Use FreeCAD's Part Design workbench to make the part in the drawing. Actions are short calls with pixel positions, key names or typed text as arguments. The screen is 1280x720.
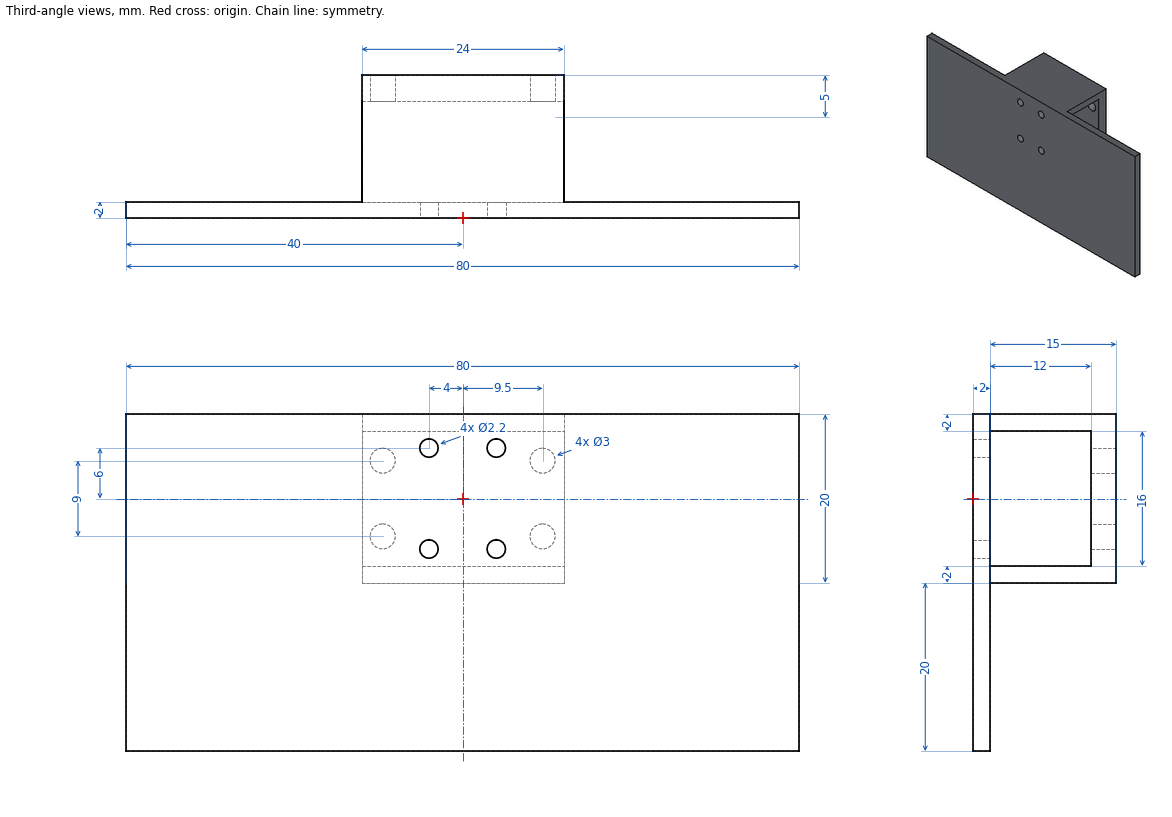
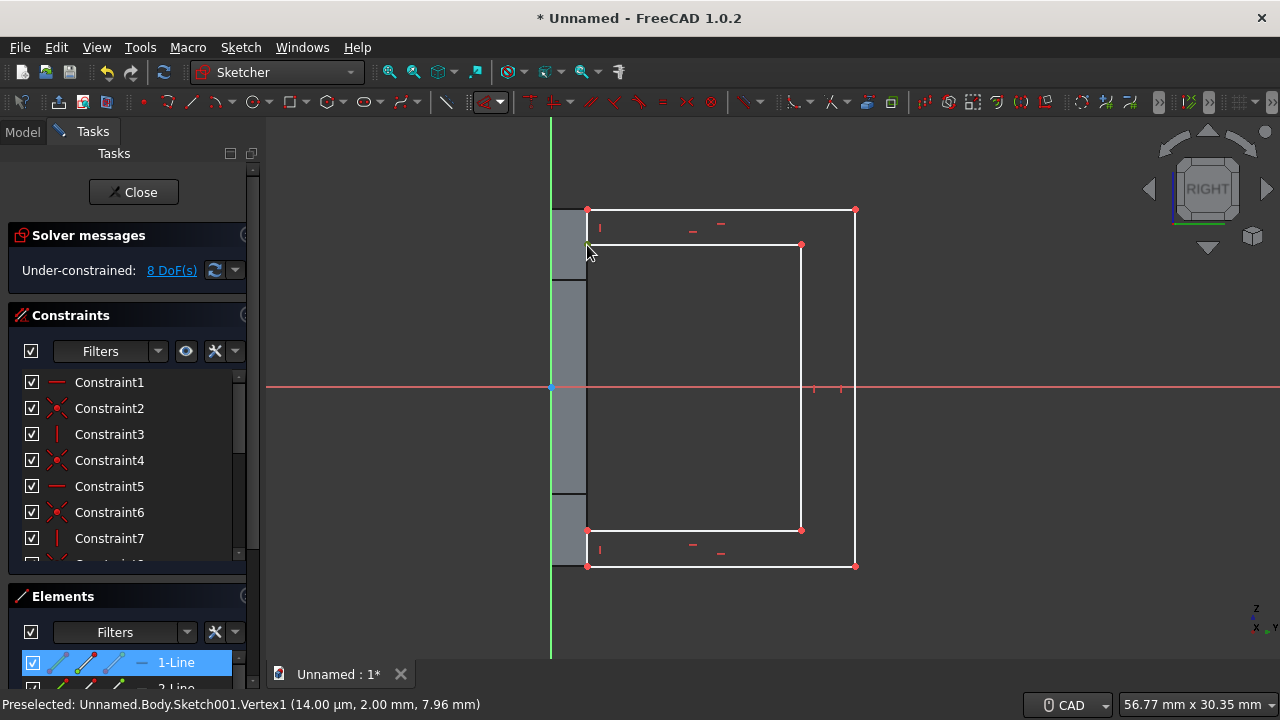
click(587, 531)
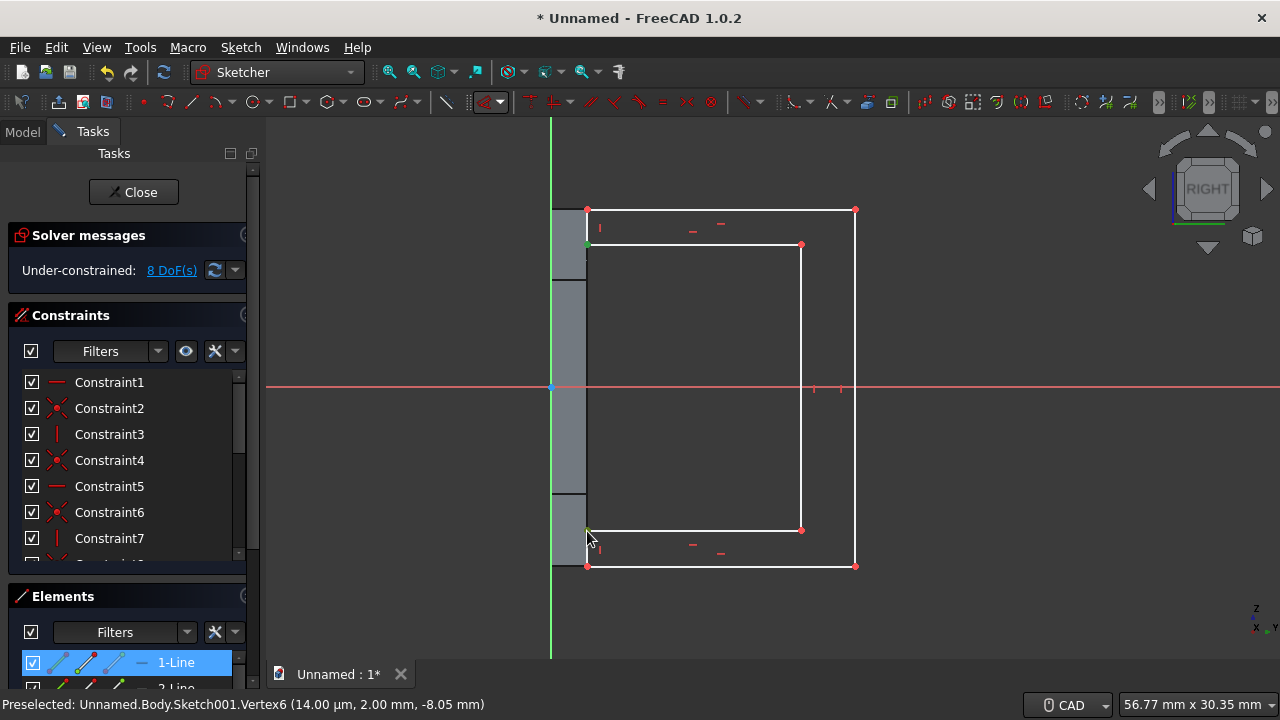
click(353, 387)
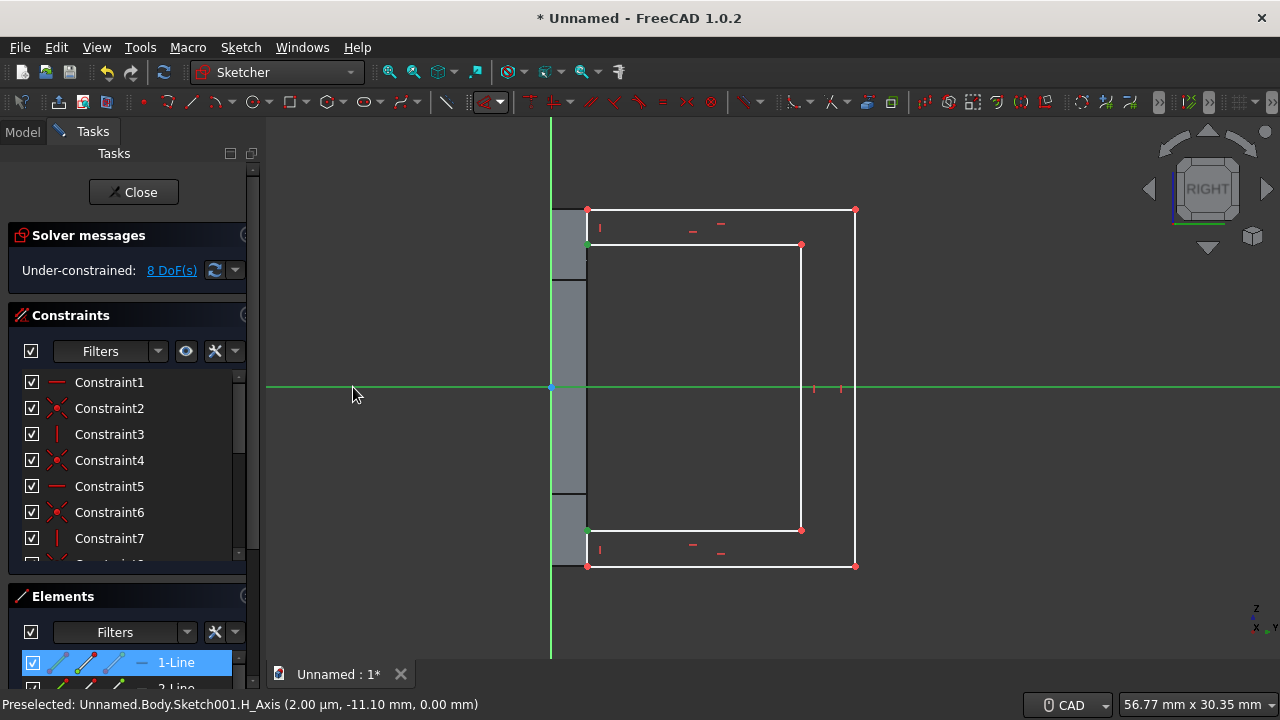
click(688, 102)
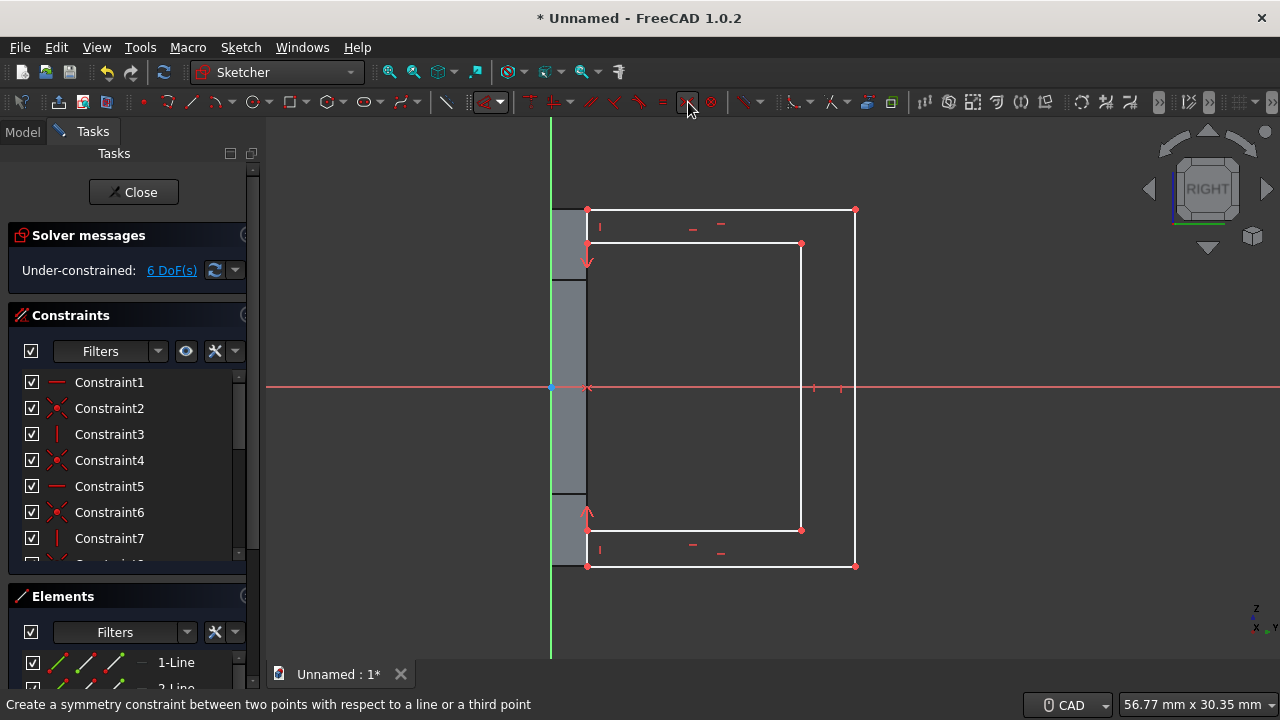
scroll(587, 542, up, 2)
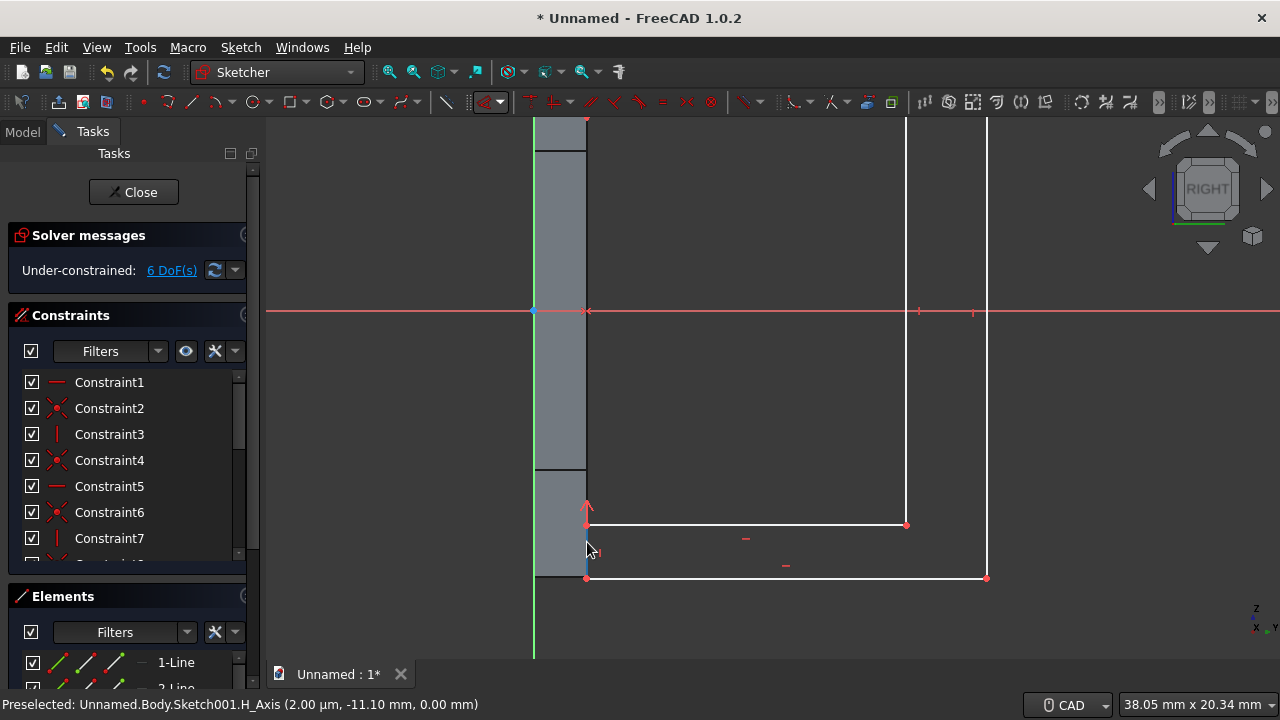
click(587, 541)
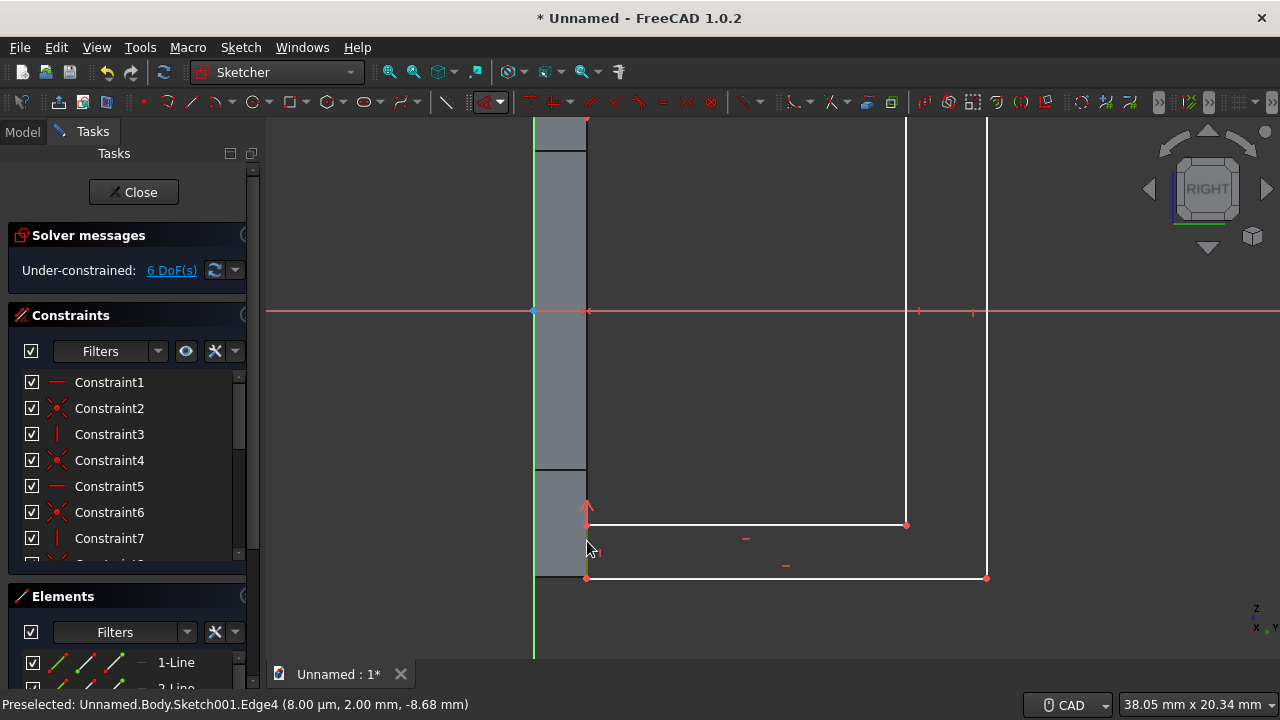
click(502, 102)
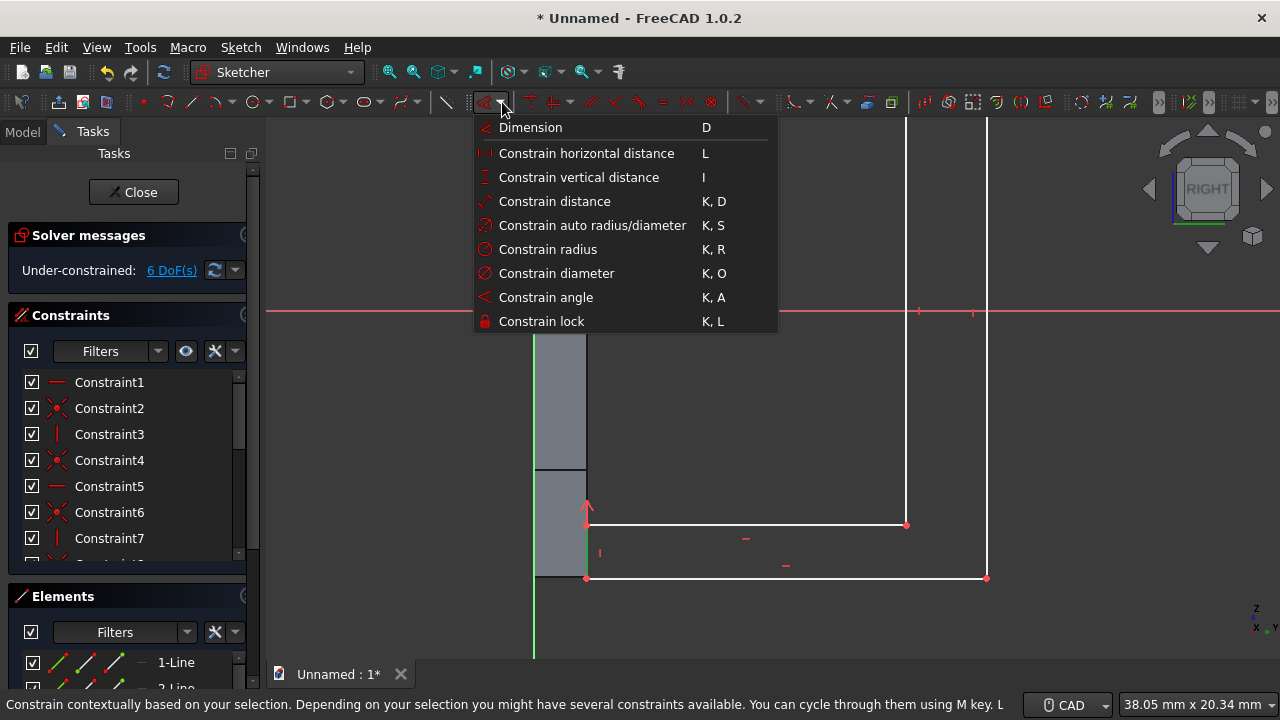
click(626, 177)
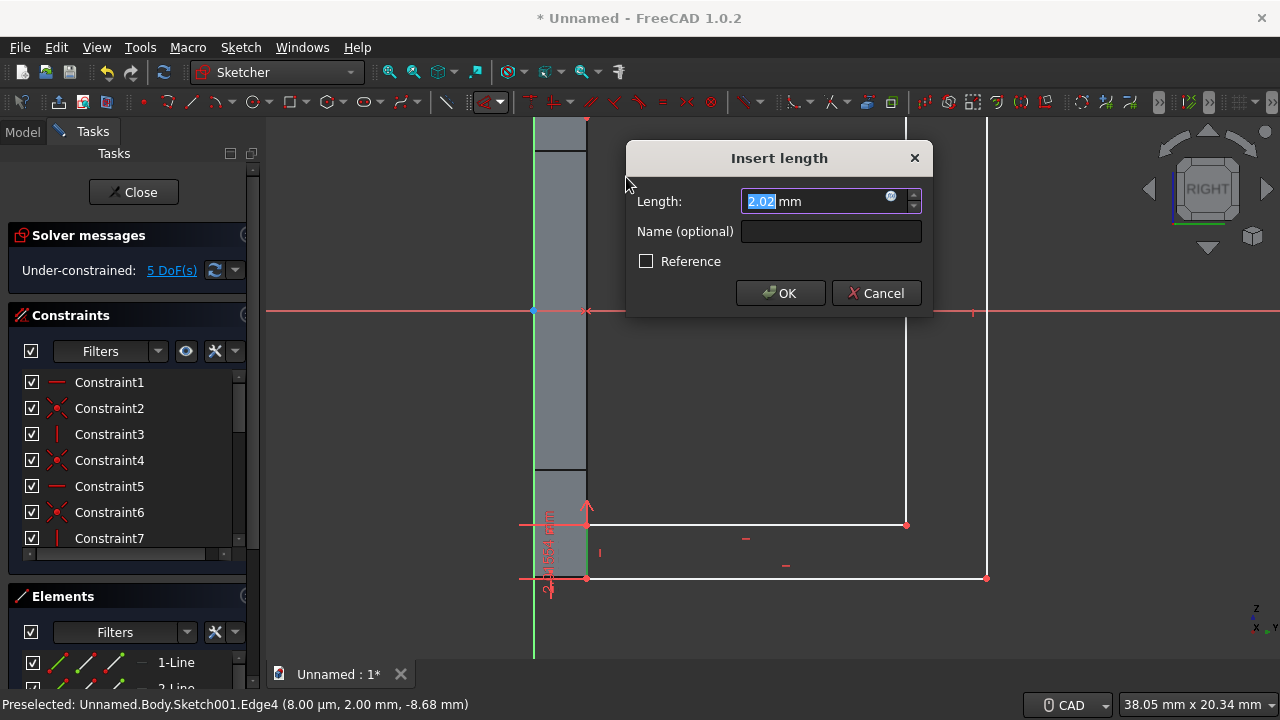
text(2)
key(Return)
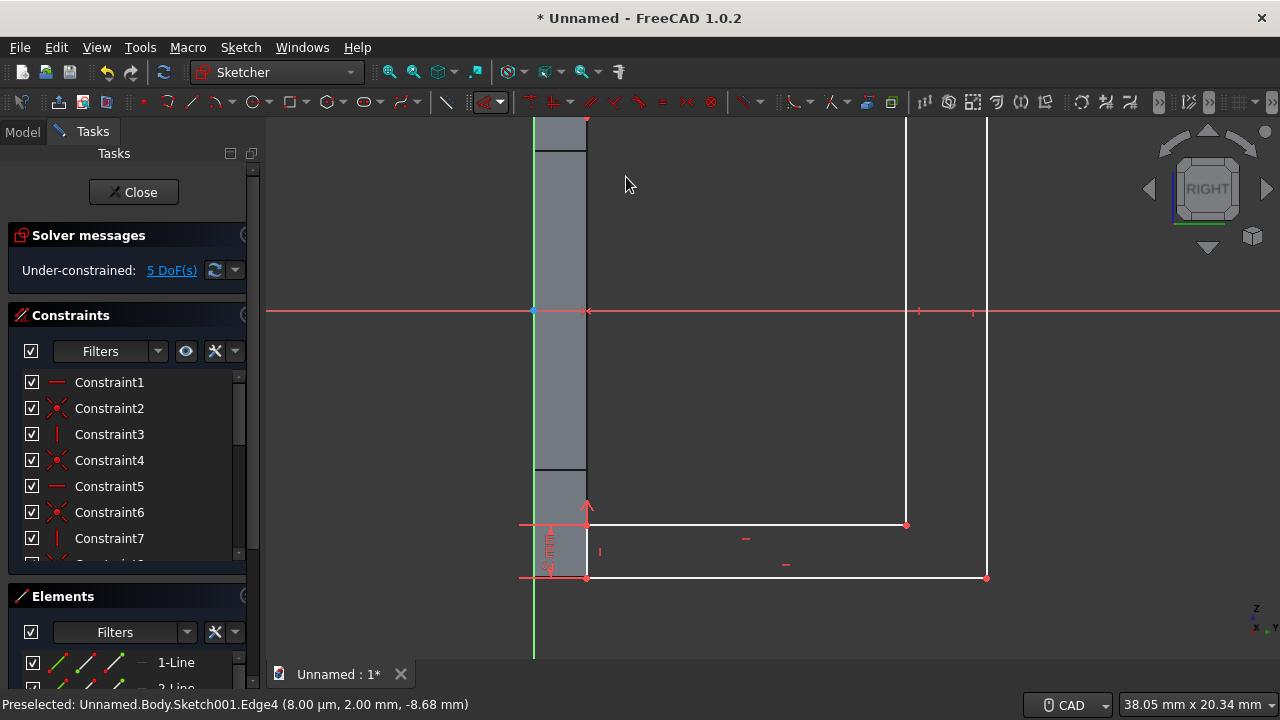
scroll(591, 545, down, 2)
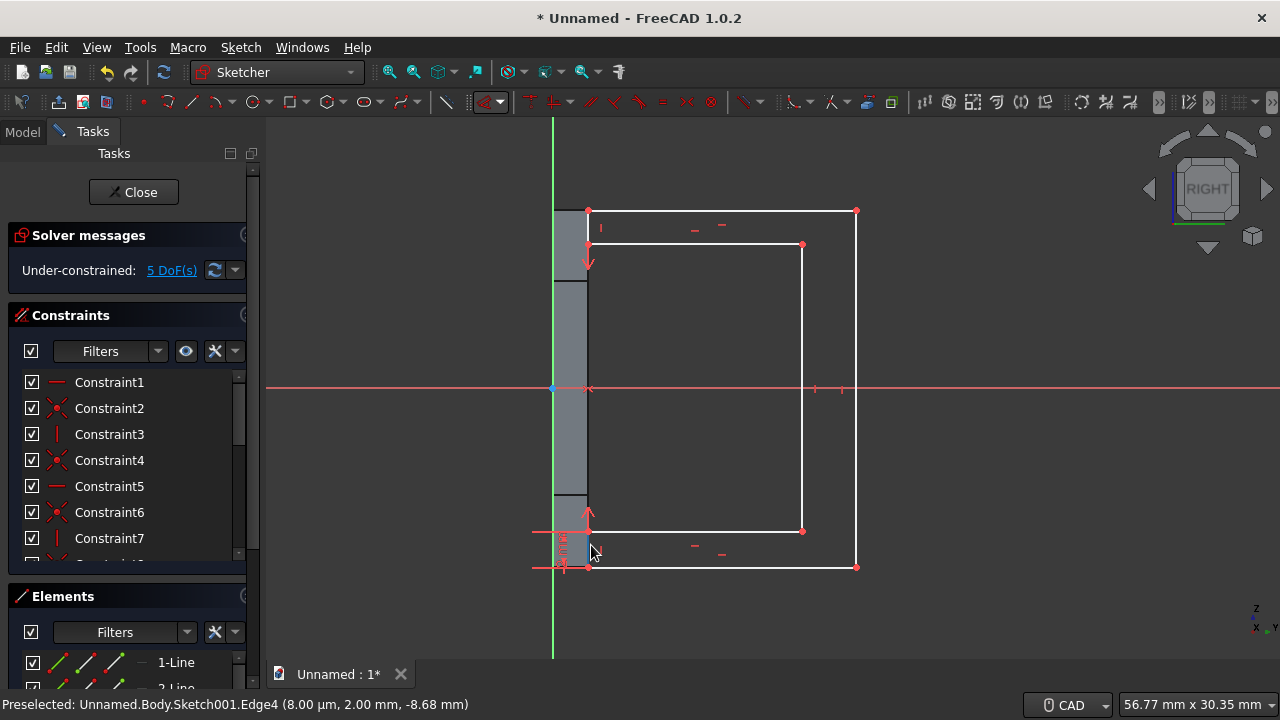
scroll(588, 221, up, 2)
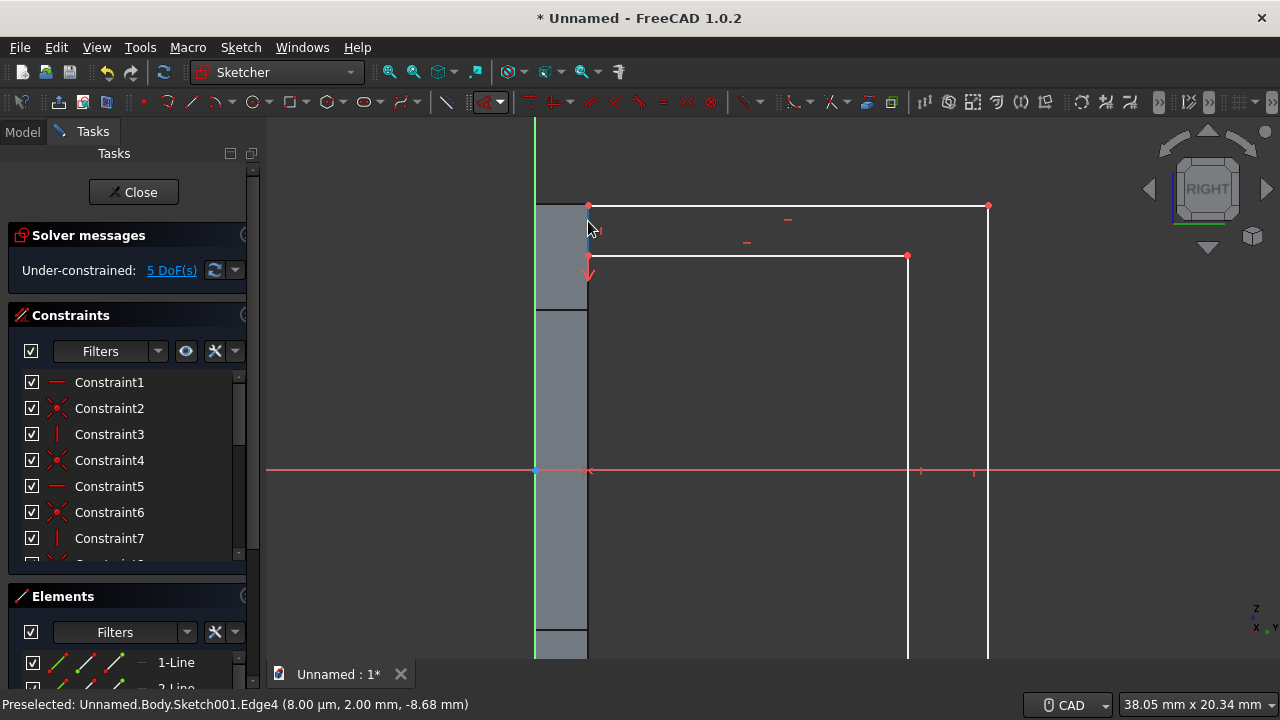
click(588, 221)